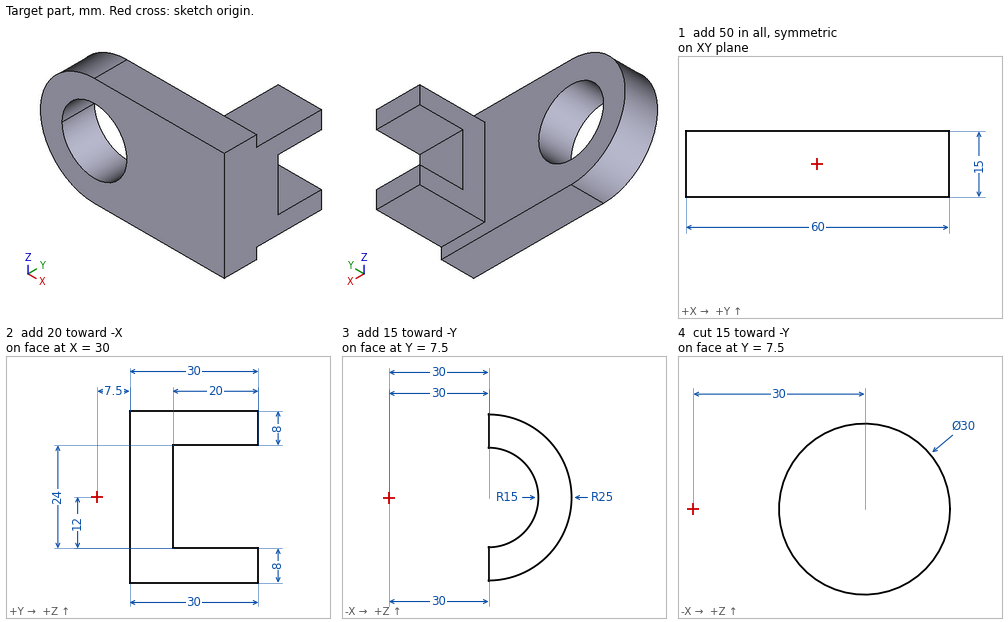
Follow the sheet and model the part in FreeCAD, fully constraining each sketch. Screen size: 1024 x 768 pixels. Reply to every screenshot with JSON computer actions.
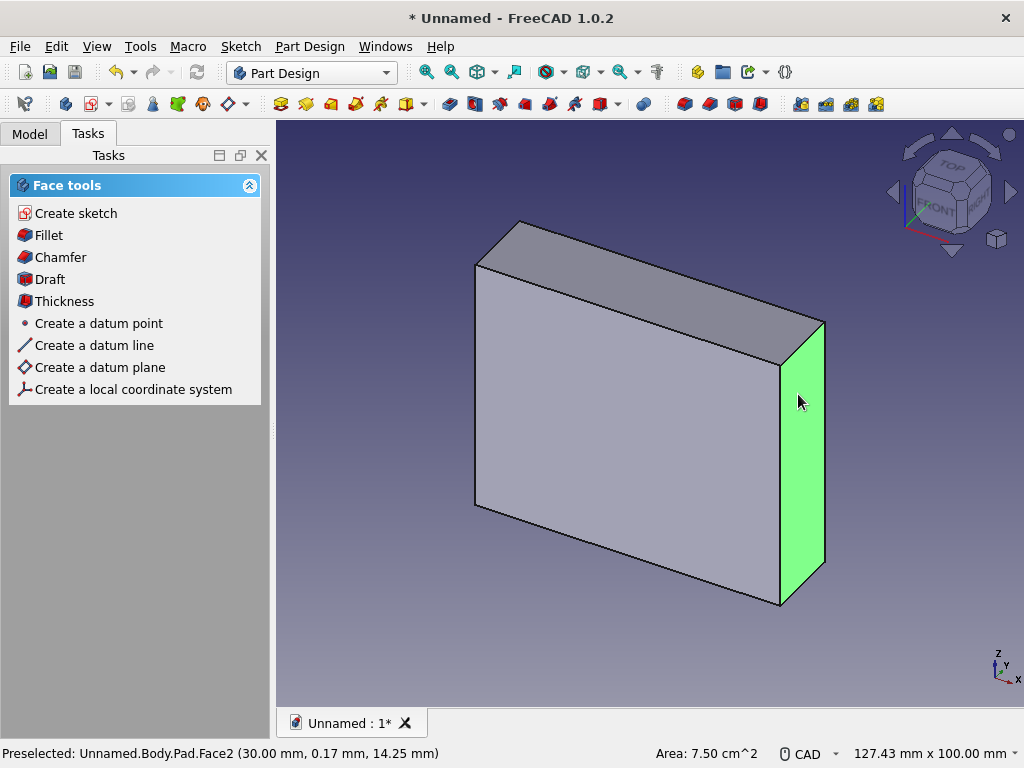
{"action": "left_click", "coordinate": [90, 104]}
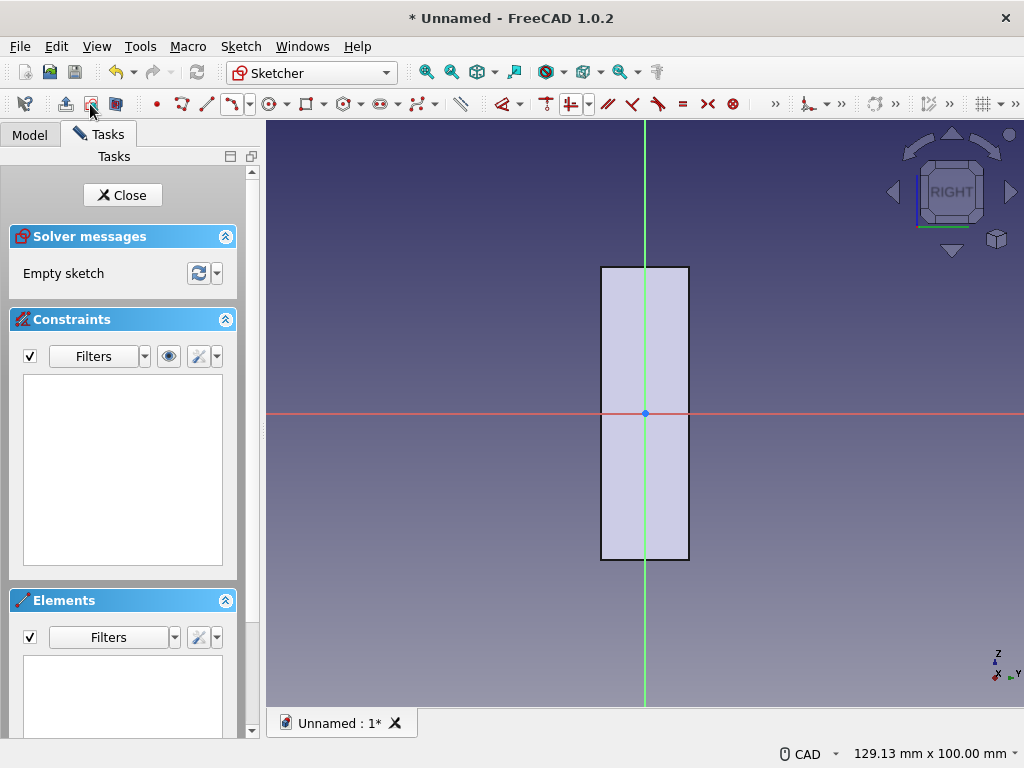
{"action": "scroll", "coordinate": [294, 413], "scroll_direction": "down", "scroll_amount": 1}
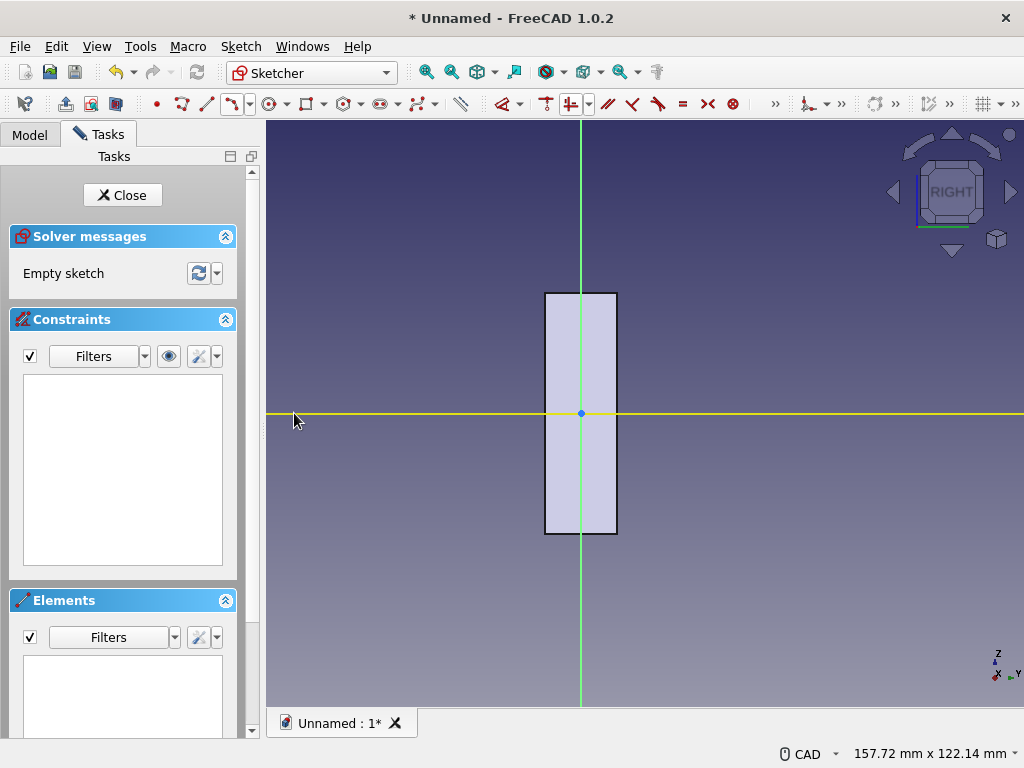
{"action": "scroll", "coordinate": [787, 414], "scroll_direction": "up", "scroll_amount": 3}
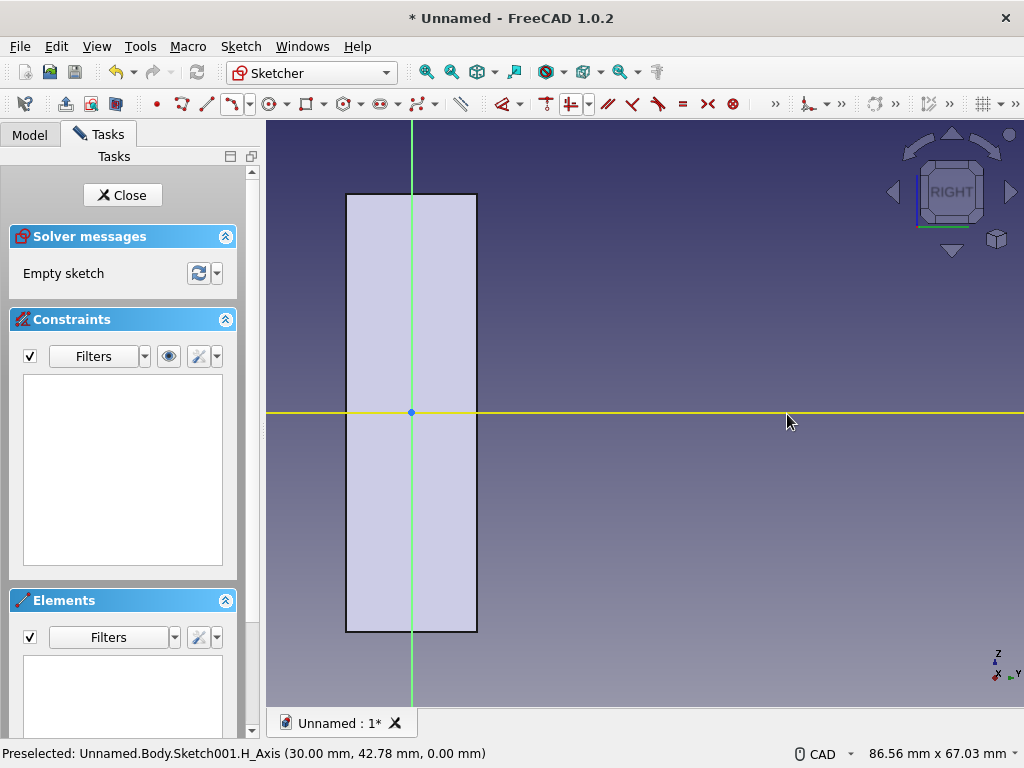
{"action": "key", "text": "g m"}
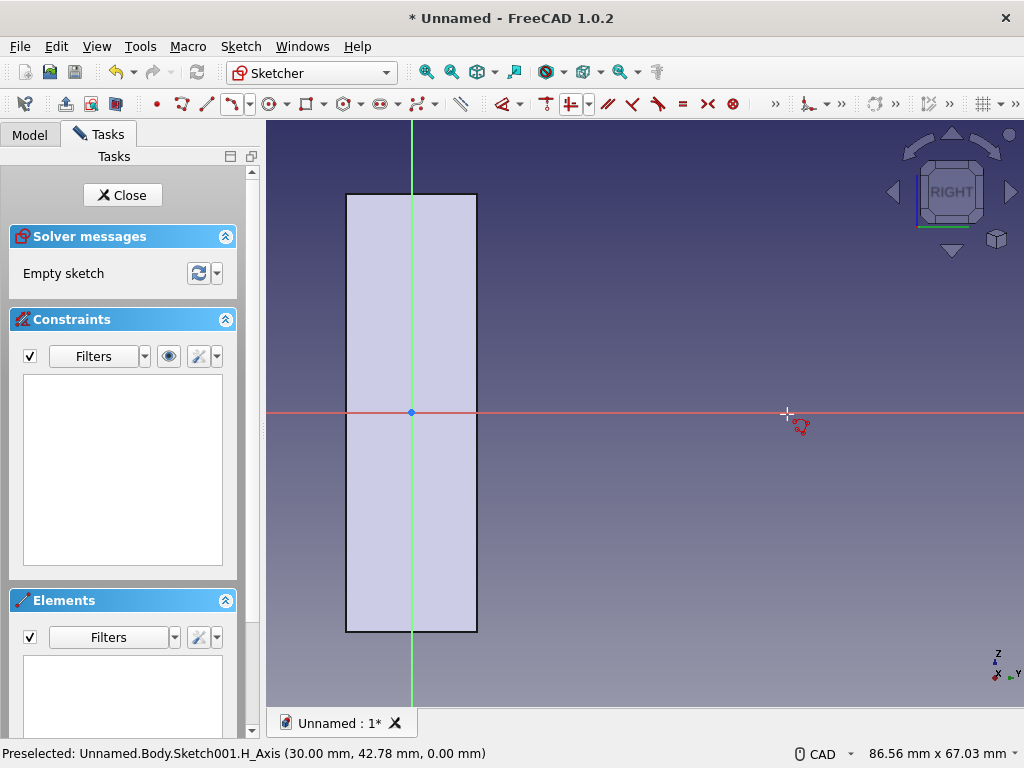
{"action": "left_click", "coordinate": [565, 518]}
{"action": "left_click", "coordinate": [565, 308]}
{"action": "left_click", "coordinate": [740, 308]}
{"action": "left_click", "coordinate": [740, 238]}
{"action": "left_click", "coordinate": [477, 238]}
{"action": "left_click", "coordinate": [477, 588]}
{"action": "left_click", "coordinate": [740, 588]}
{"action": "left_click", "coordinate": [740, 518]}
{"action": "left_click", "coordinate": [565, 519]}
{"action": "key", "text": "Escape"}
{"action": "key", "text": "Escape"}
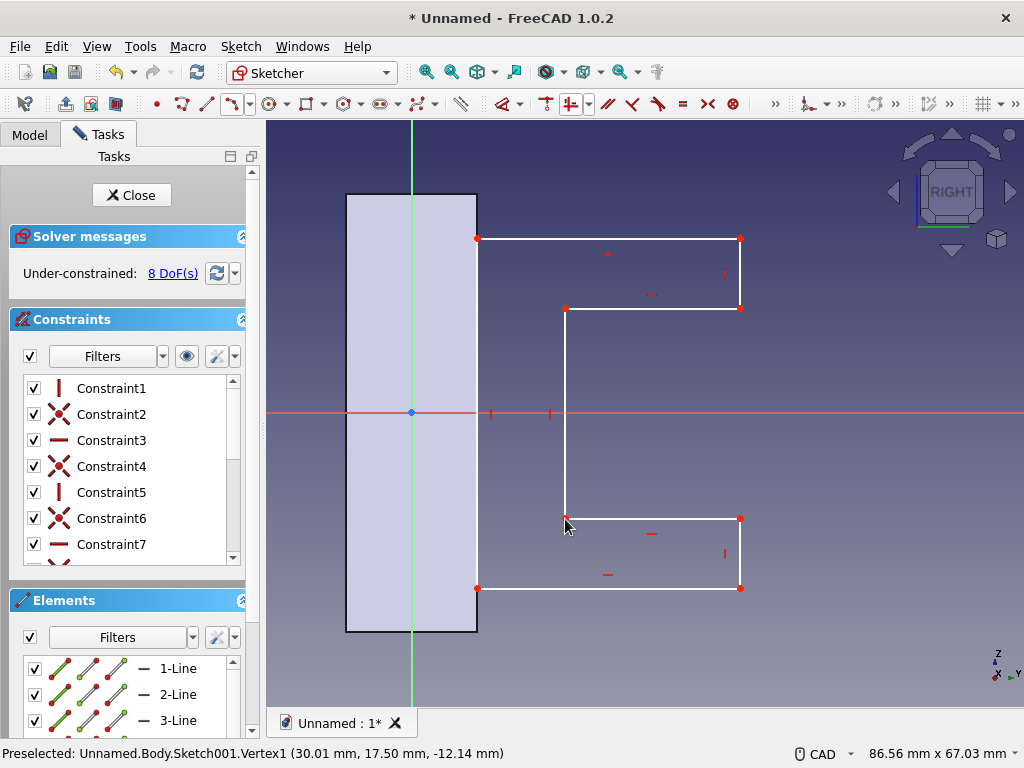
{"action": "key", "text": "d"}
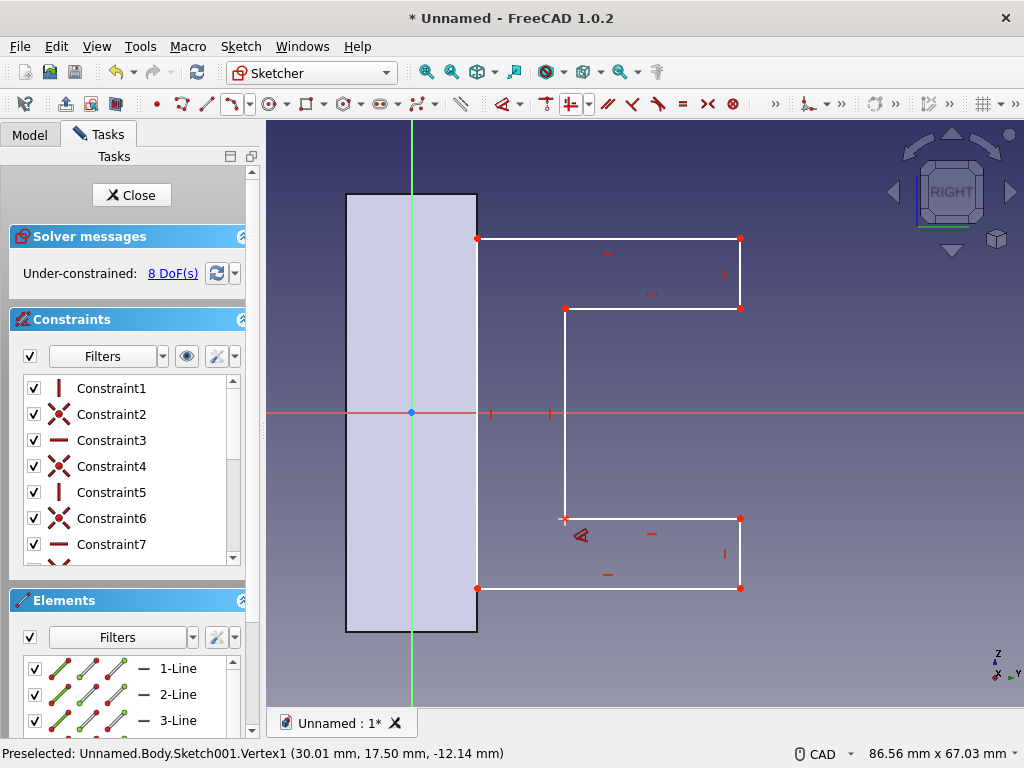
{"action": "left_click", "coordinate": [740, 288]}
{"action": "left_click", "coordinate": [774, 274]}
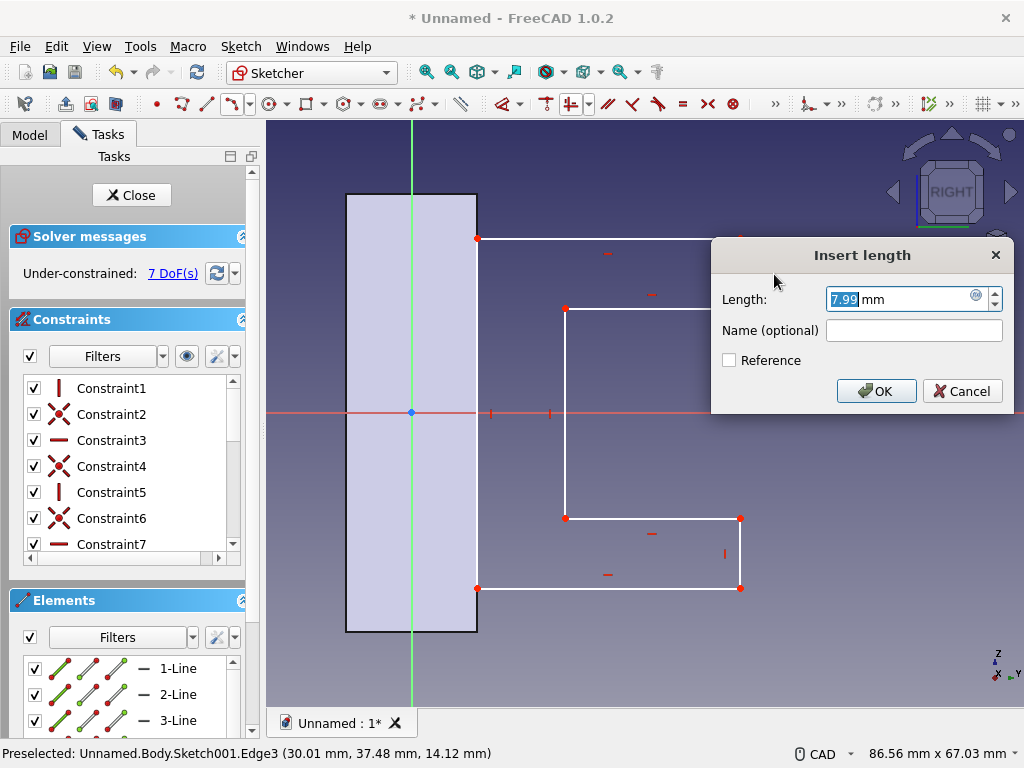
{"action": "type", "text": "8"}
{"action": "key", "text": "Return"}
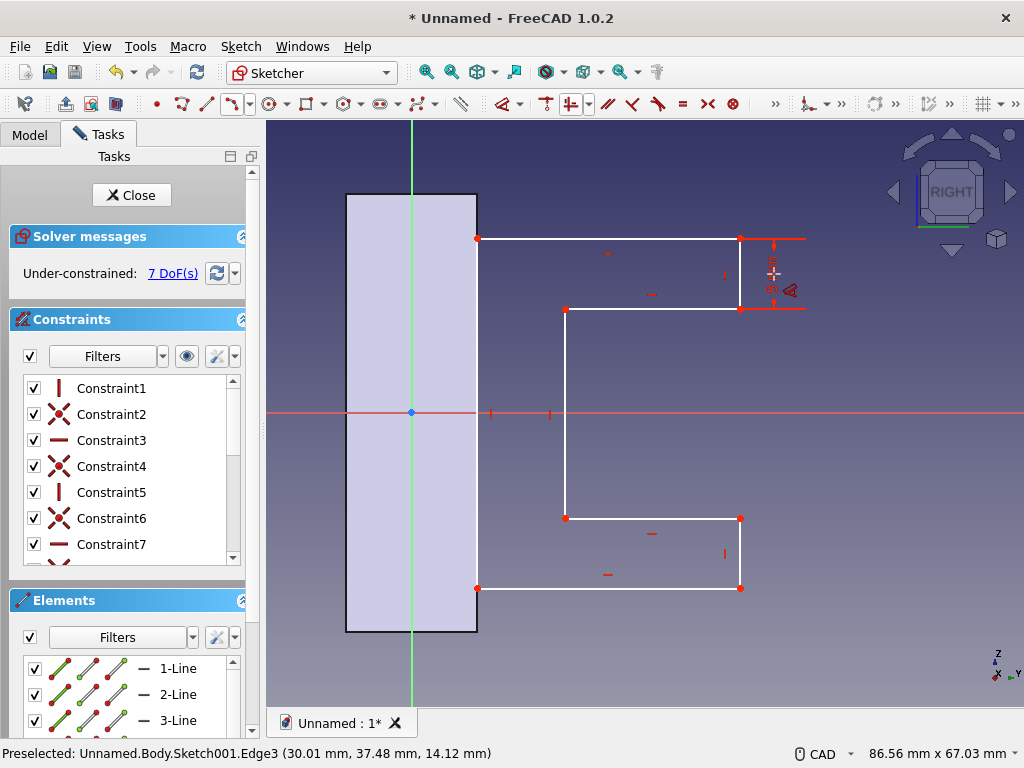
{"action": "left_click", "coordinate": [740, 568]}
{"action": "left_click", "coordinate": [774, 554]}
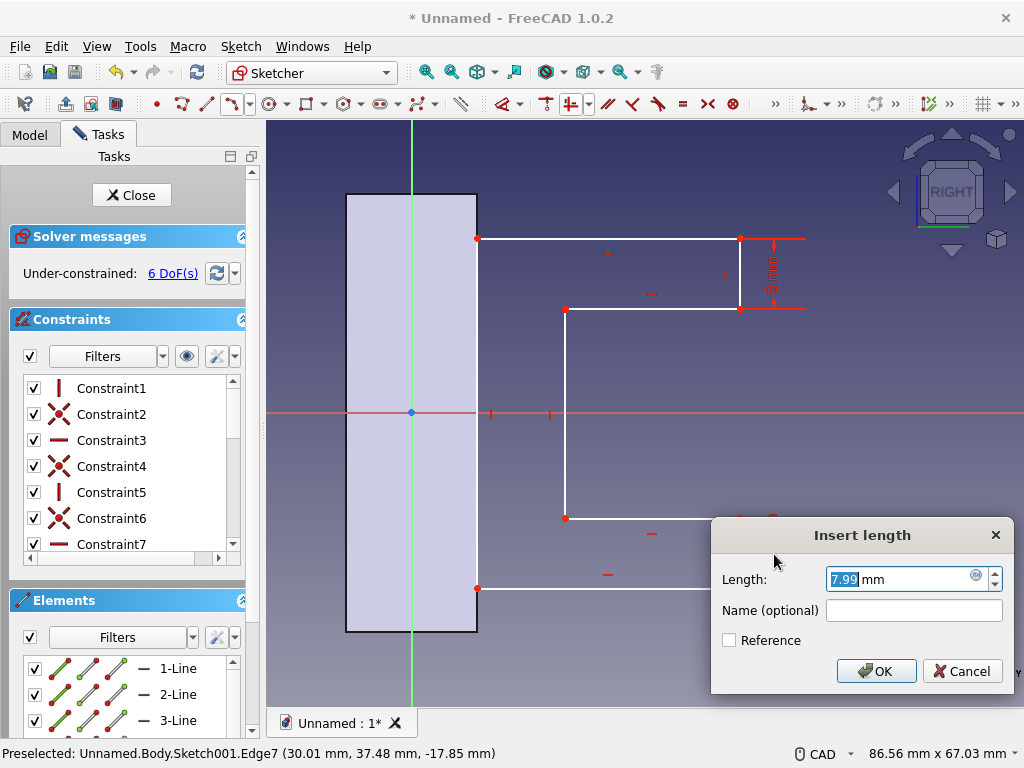
{"action": "type", "text": "8"}
{"action": "key", "text": "Return"}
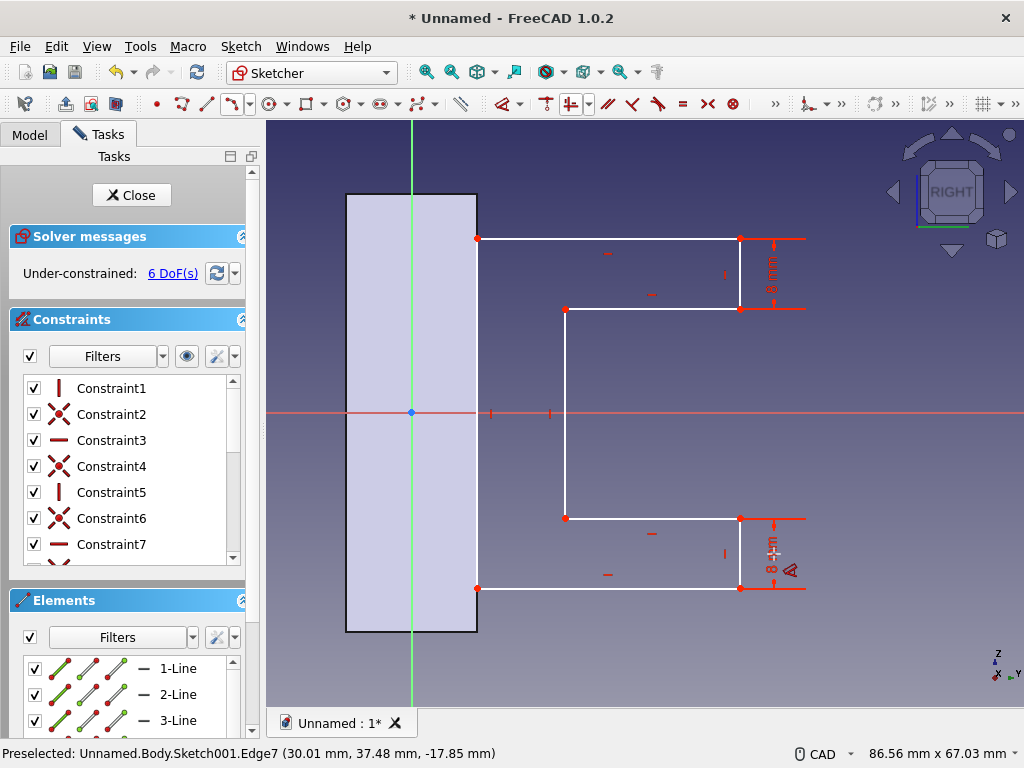
{"action": "left_click", "coordinate": [565, 456]}
{"action": "left_click", "coordinate": [531, 366]}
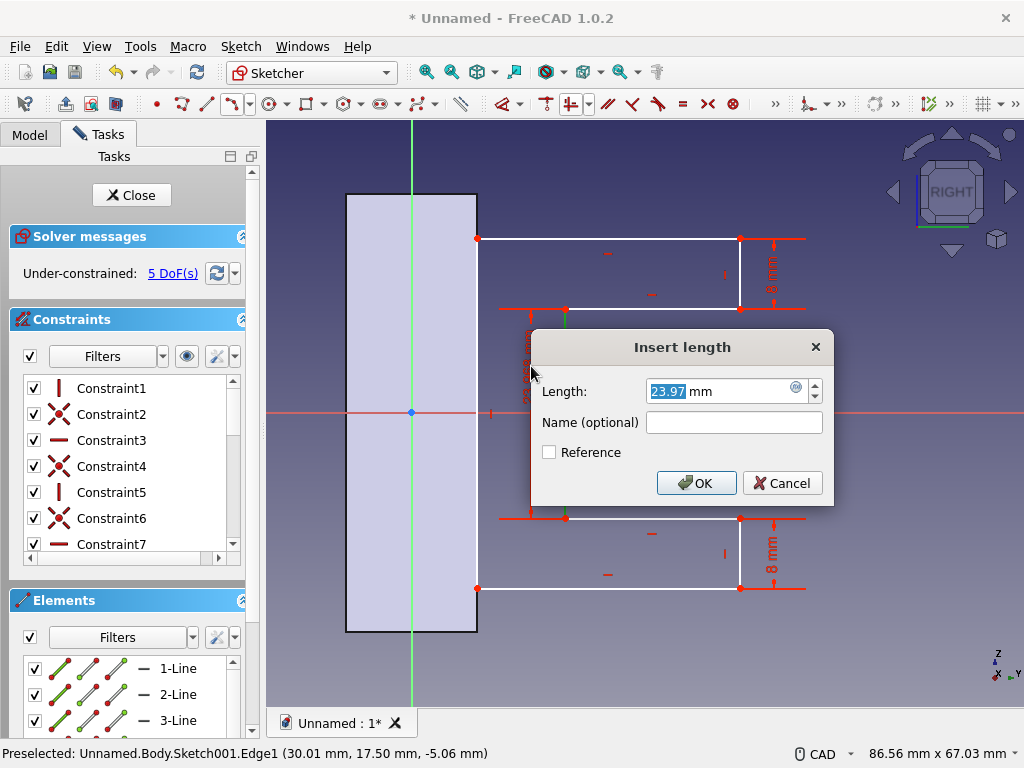
{"action": "type", "text": "24"}
{"action": "key", "text": "Return"}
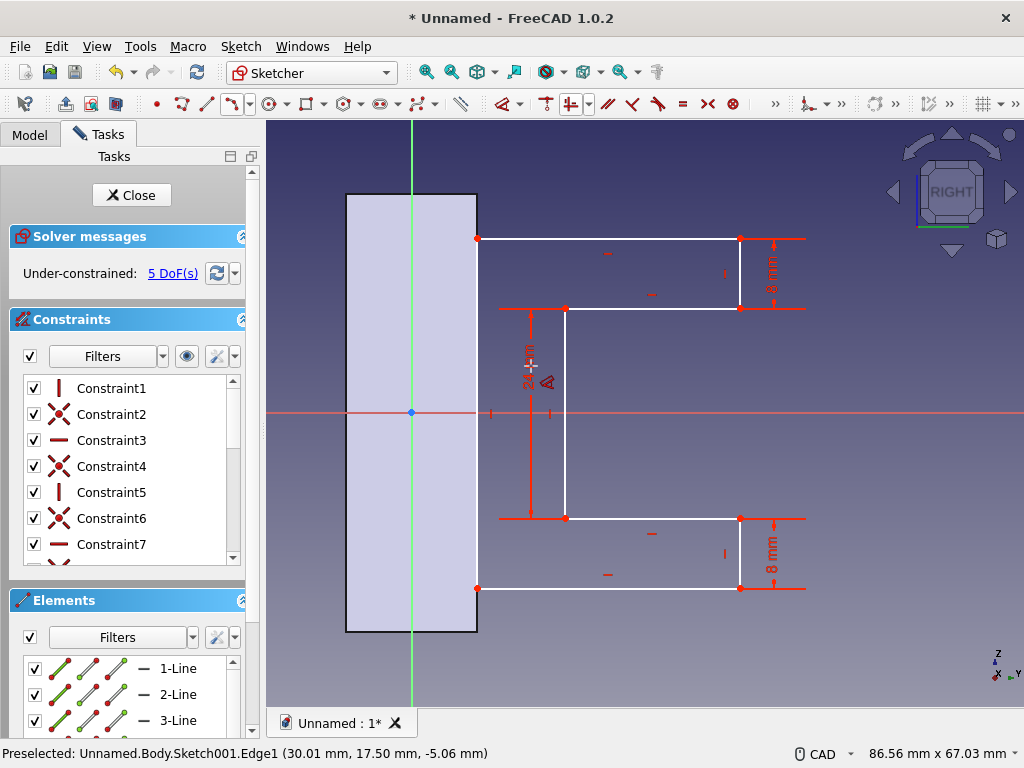
{"action": "left_click", "coordinate": [617, 309]}
{"action": "left_click", "coordinate": [652, 275]}